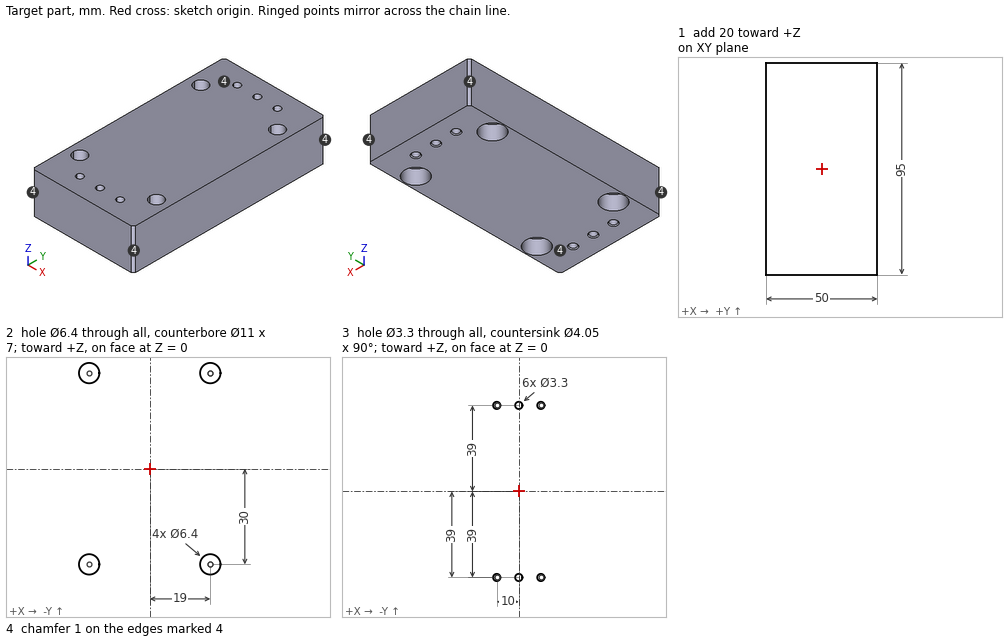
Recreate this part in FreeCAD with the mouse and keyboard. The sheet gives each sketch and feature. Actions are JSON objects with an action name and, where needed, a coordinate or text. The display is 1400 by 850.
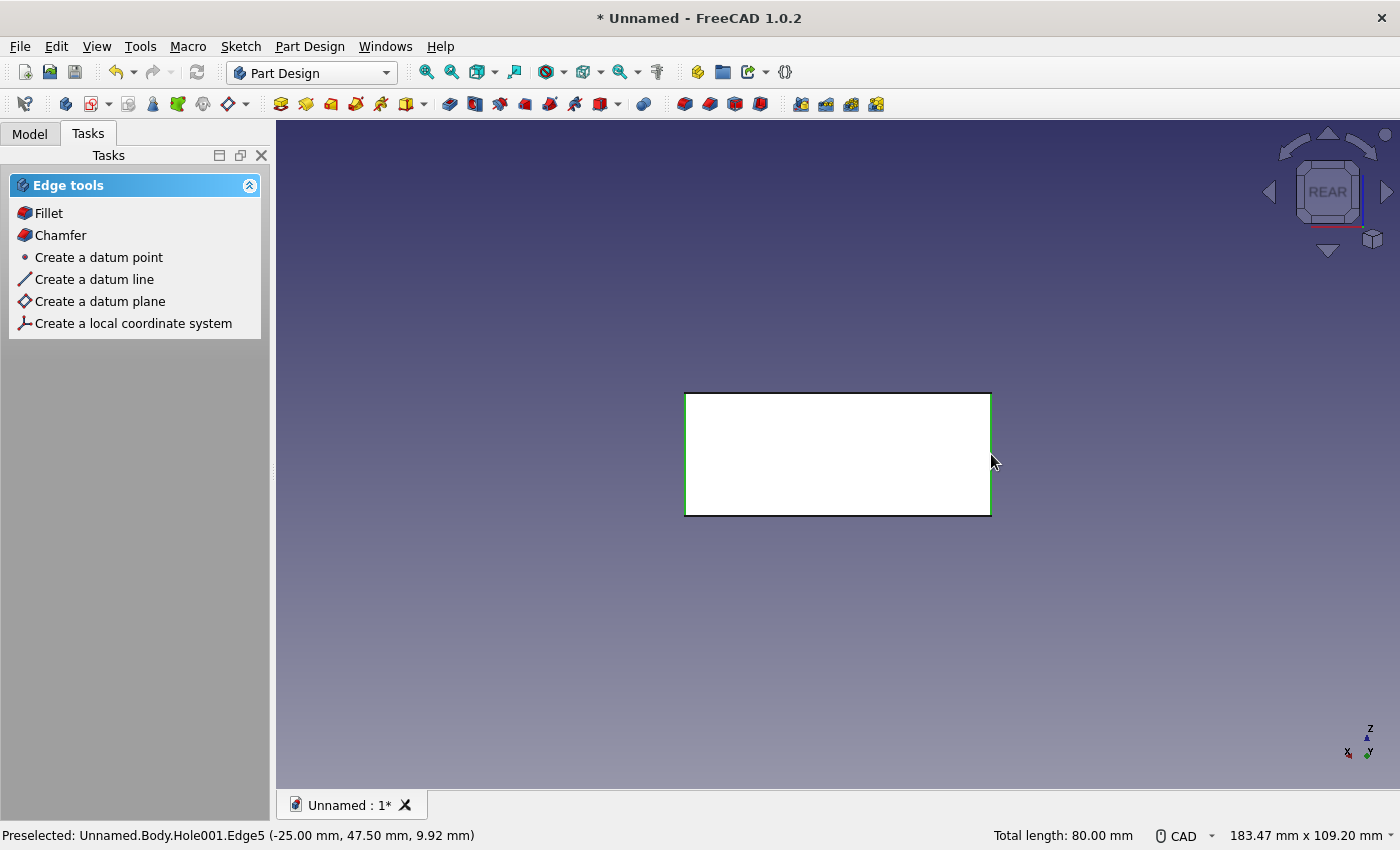
{"action": "left_click", "coordinate": [710, 104]}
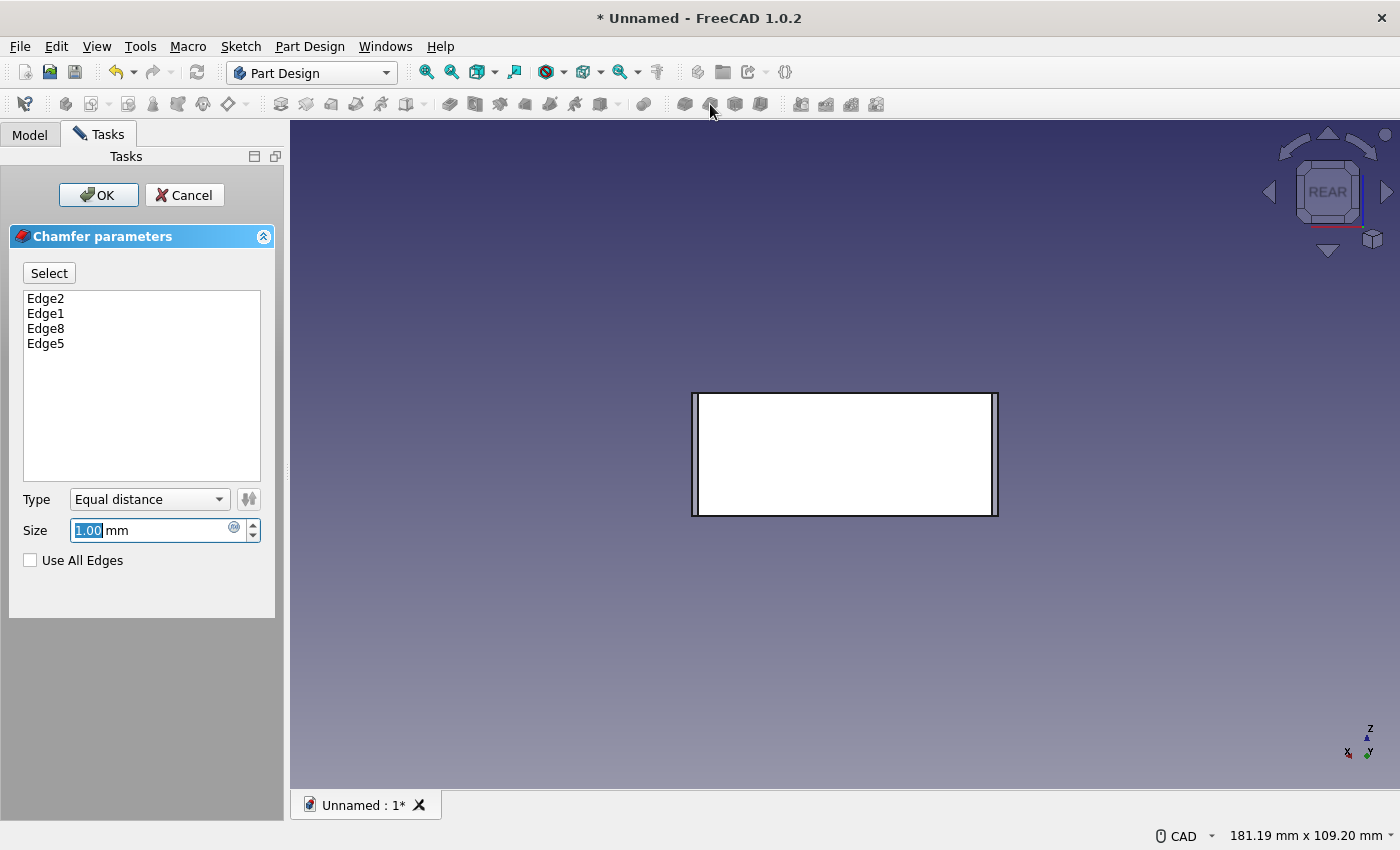
{"action": "type", "text": "1"}
{"action": "key", "text": "Tab"}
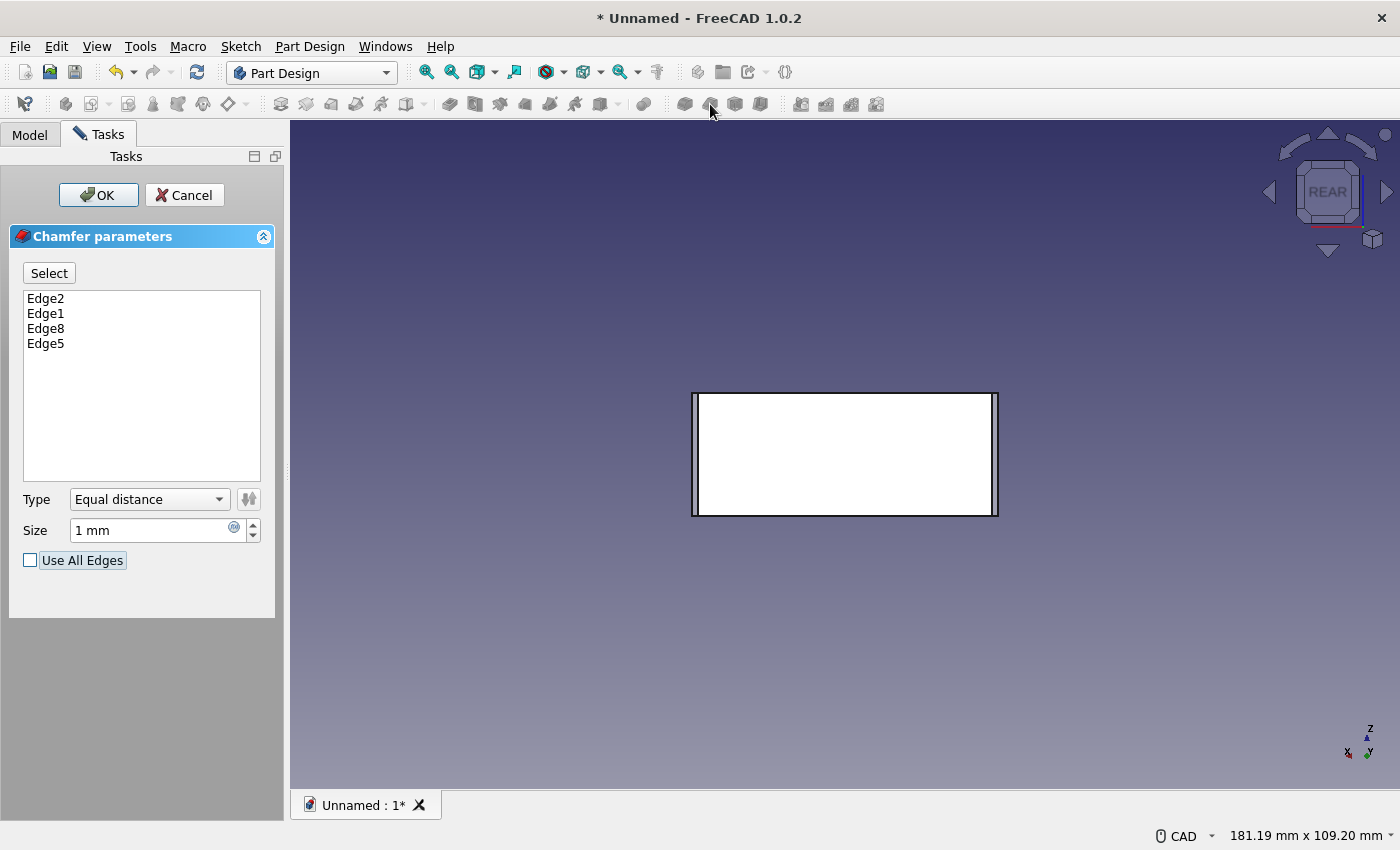
{"action": "left_click", "coordinate": [99, 195]}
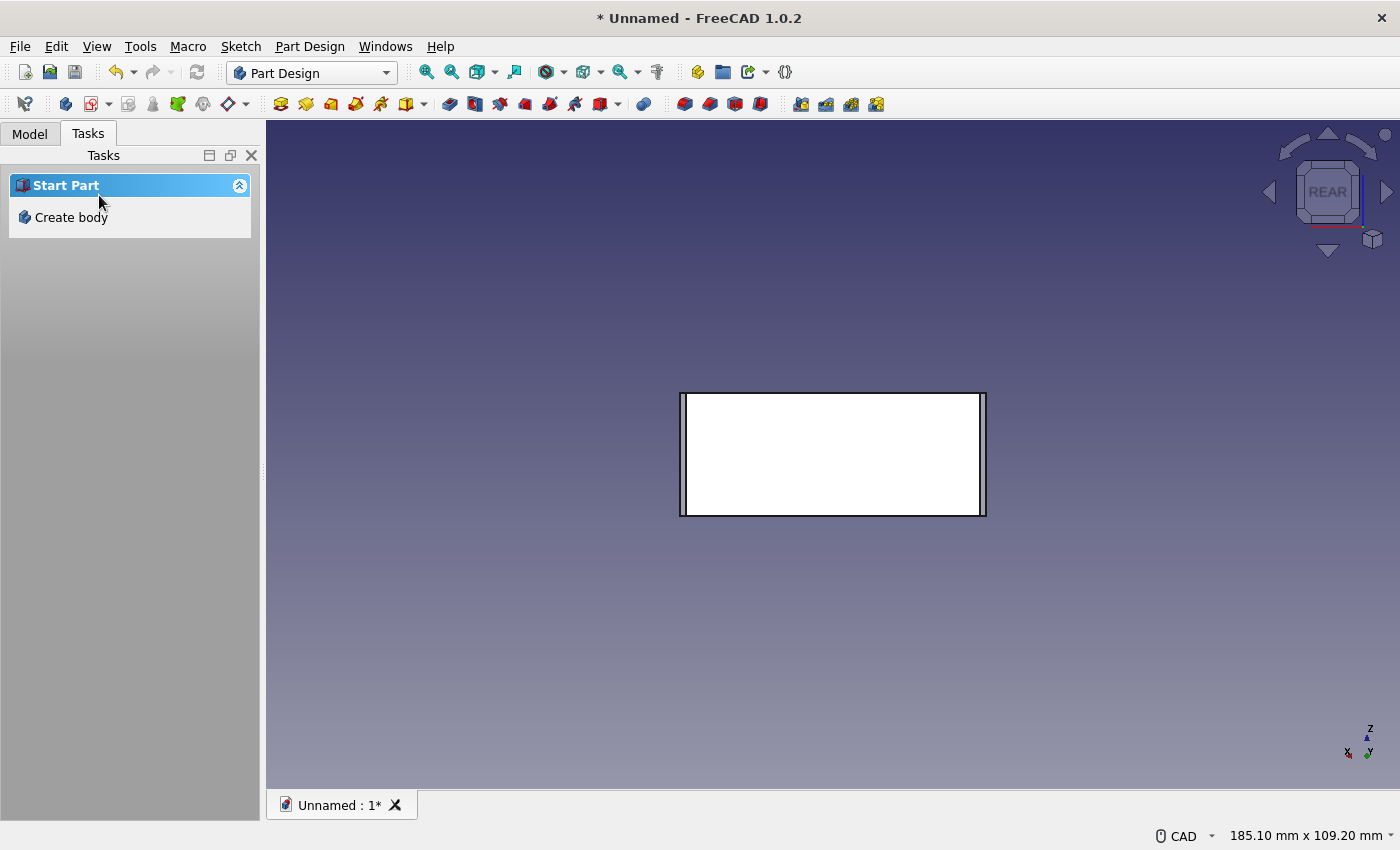
{"action": "key", "text": "0"}